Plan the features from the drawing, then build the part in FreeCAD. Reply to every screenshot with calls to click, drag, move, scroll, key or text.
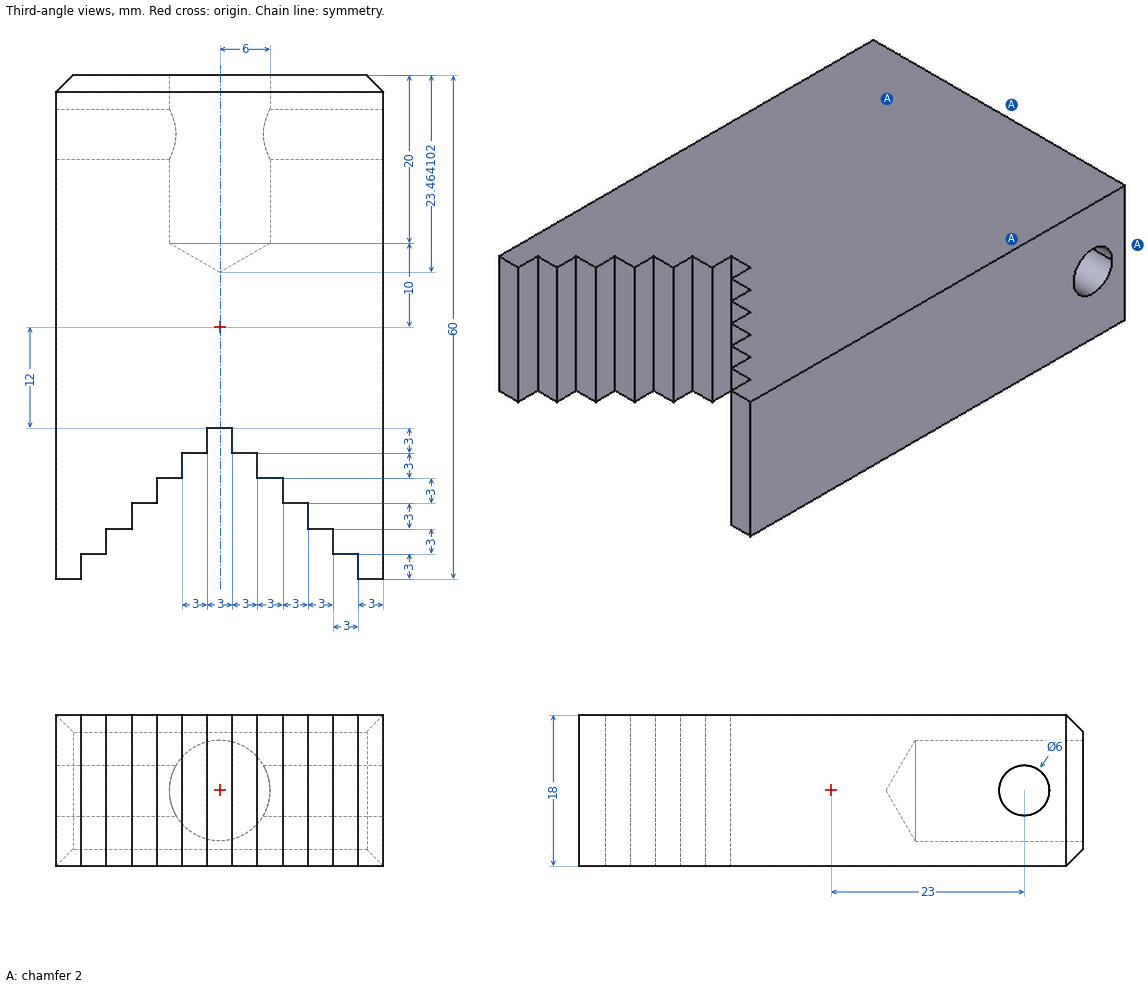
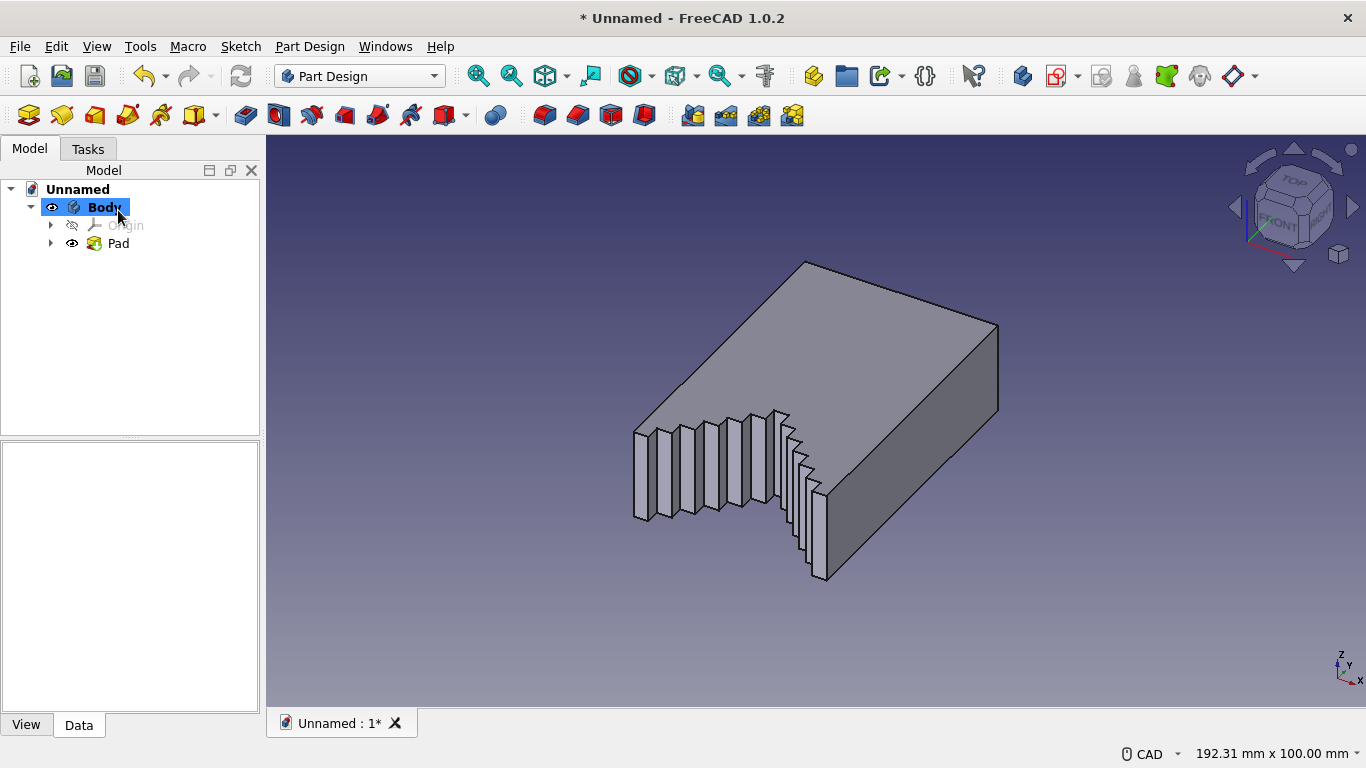
key(0)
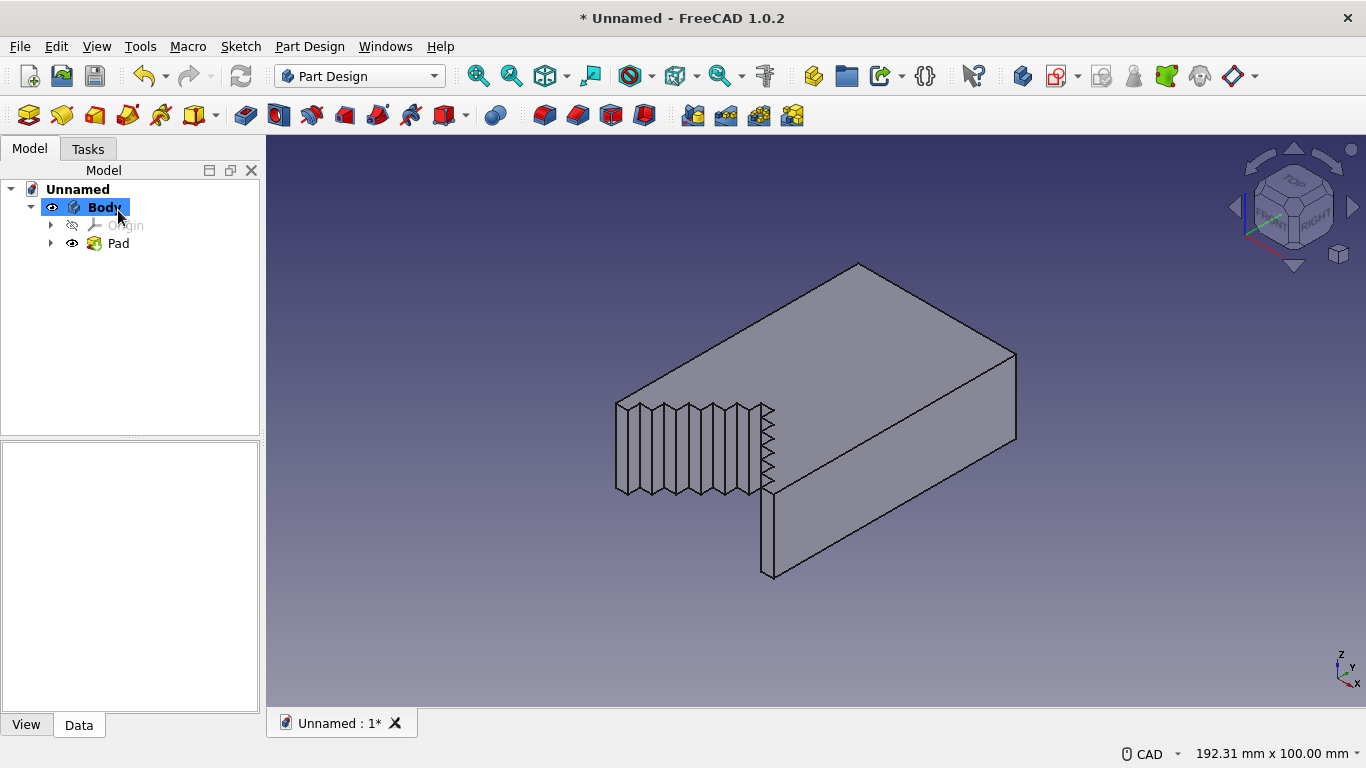
key(2)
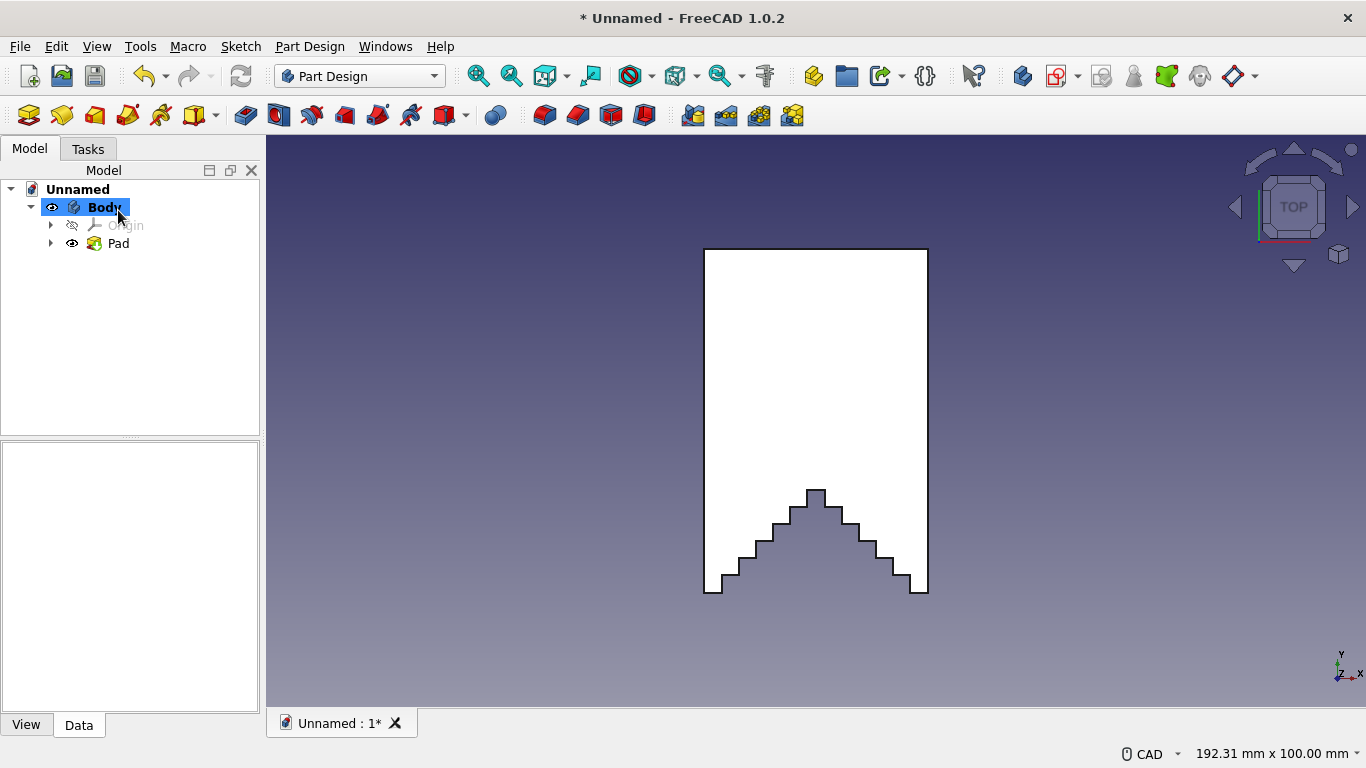
key(1)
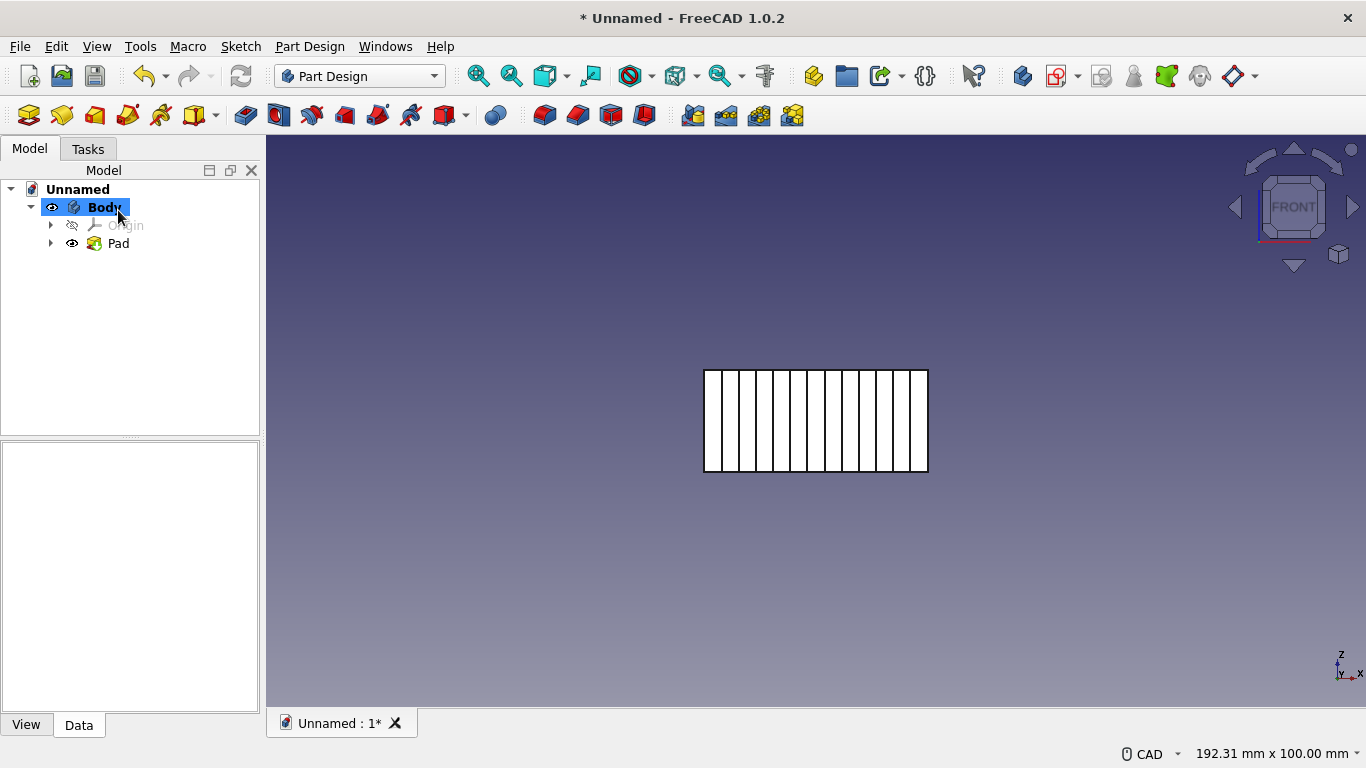
click(479, 76)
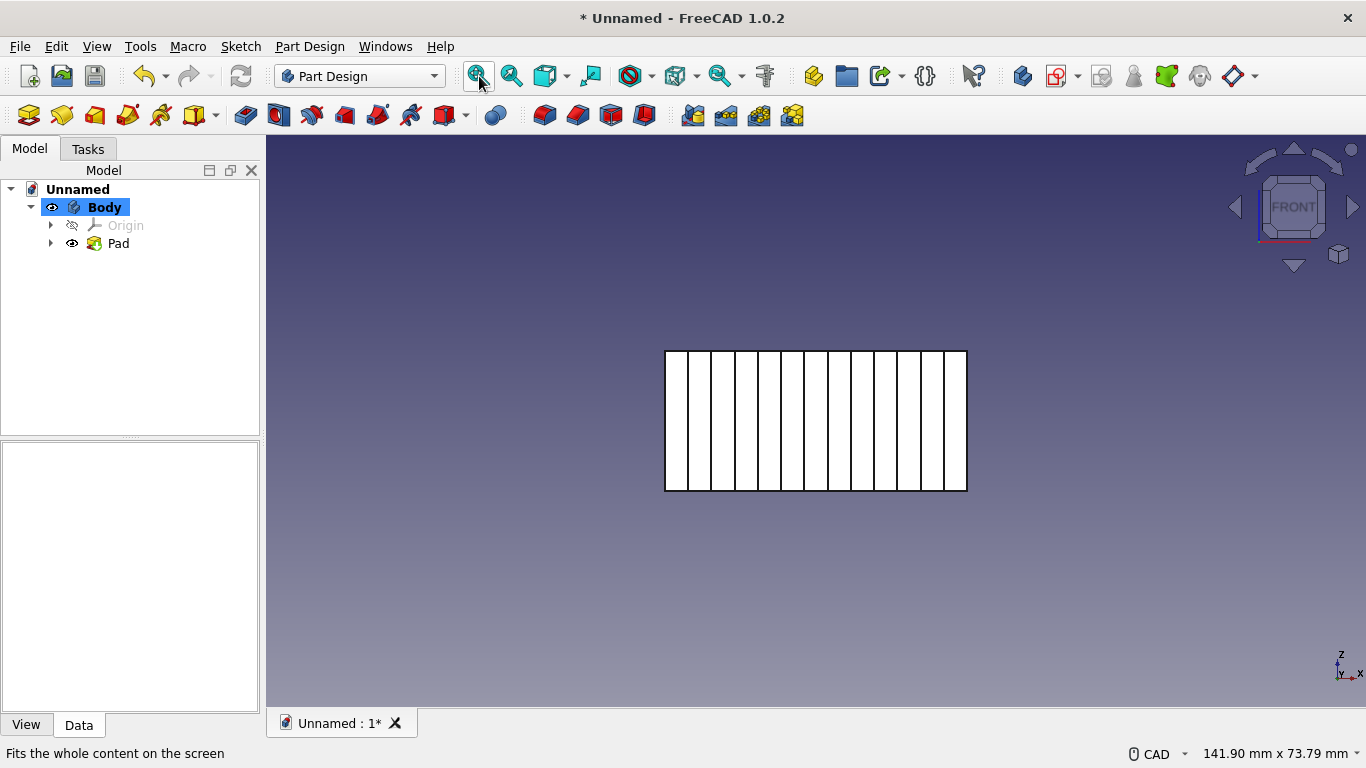
key(3)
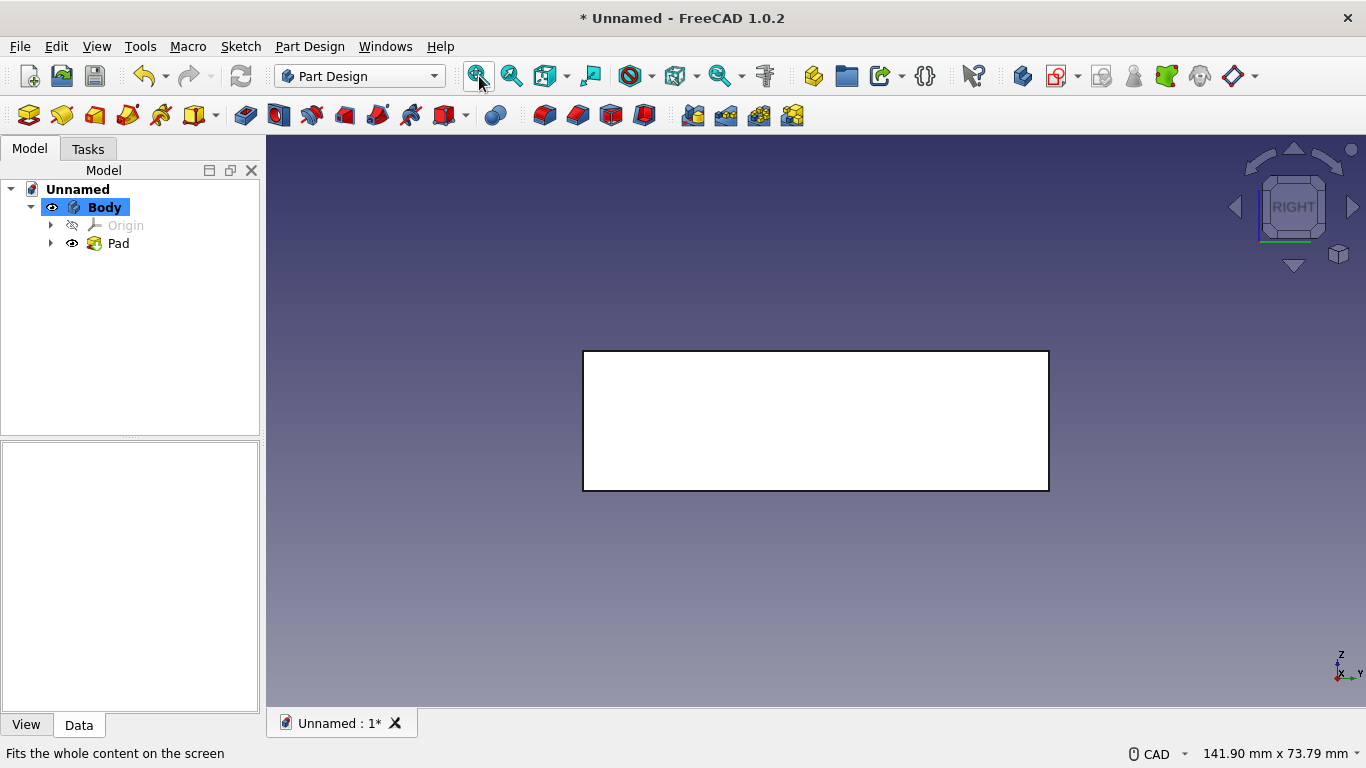
click(479, 76)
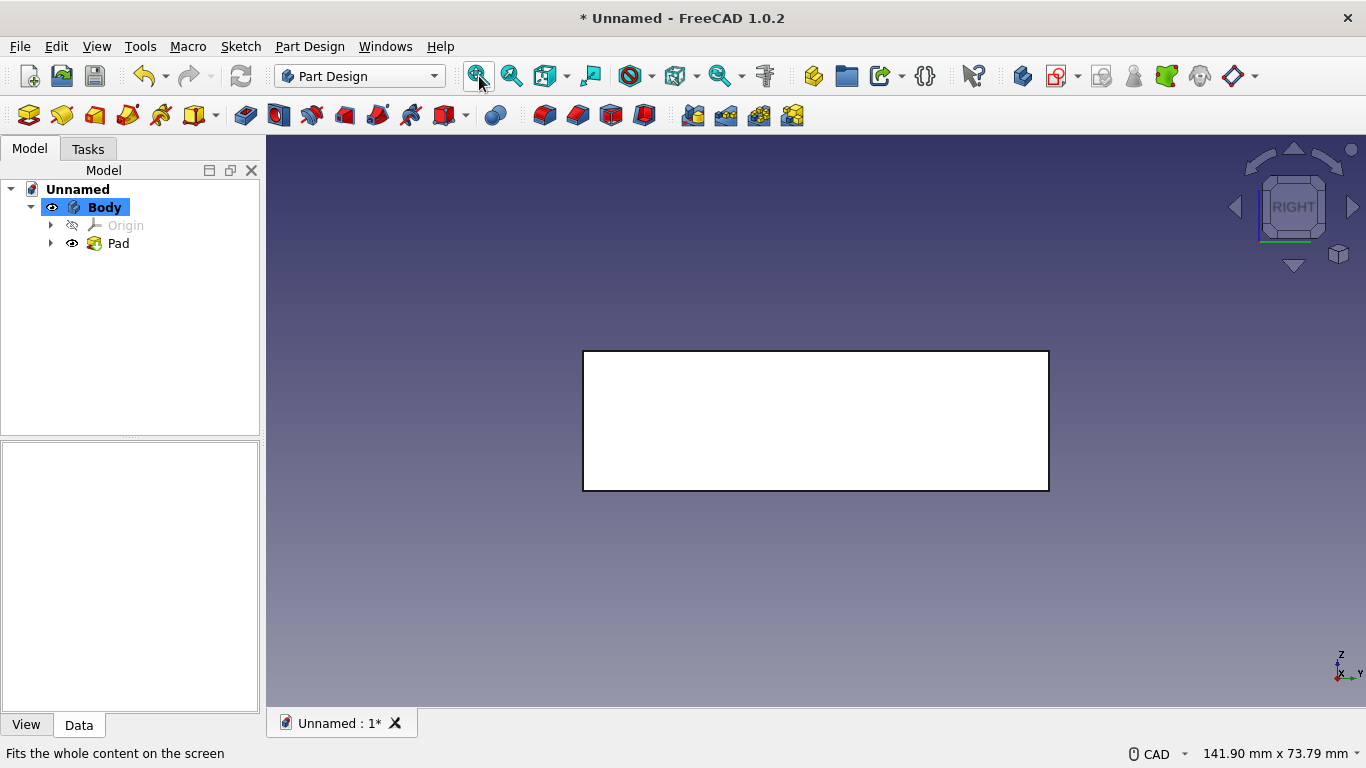
key(5)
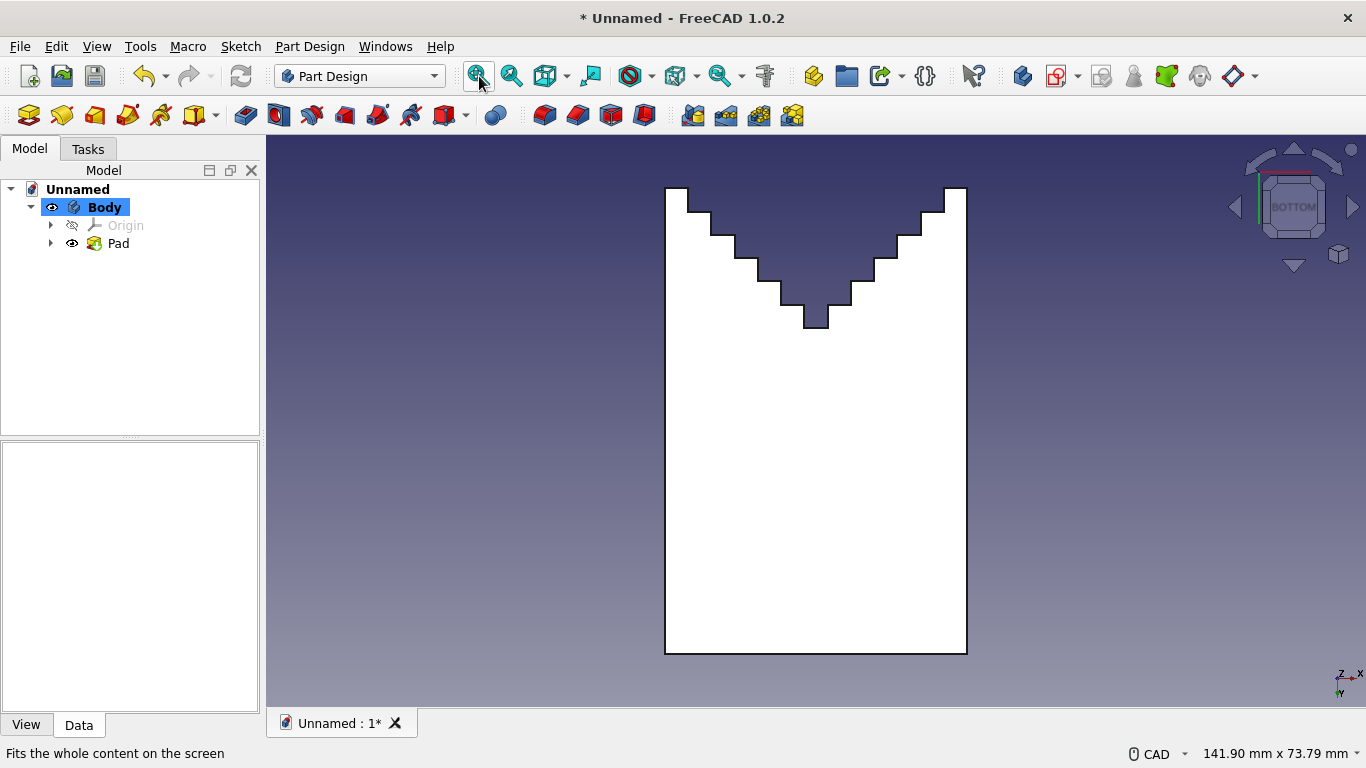
key(4)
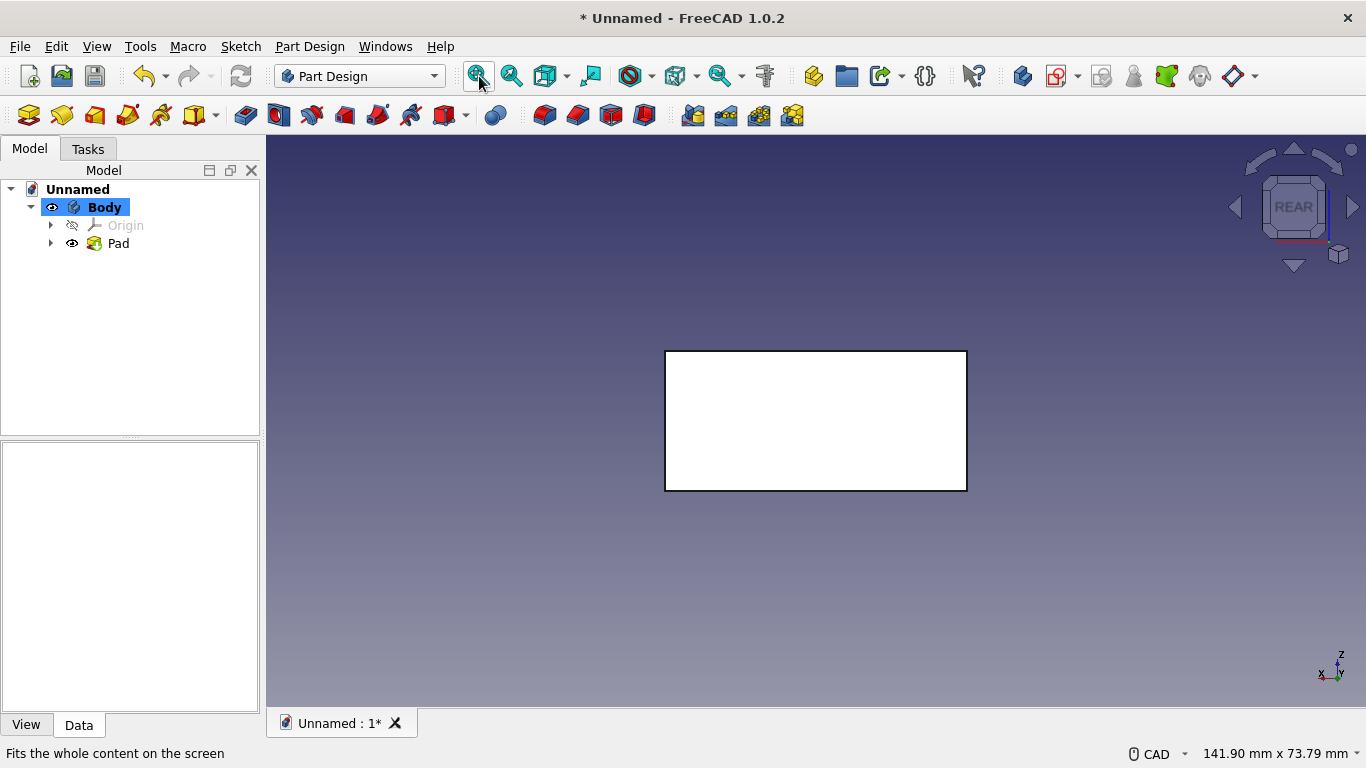
click(479, 76)